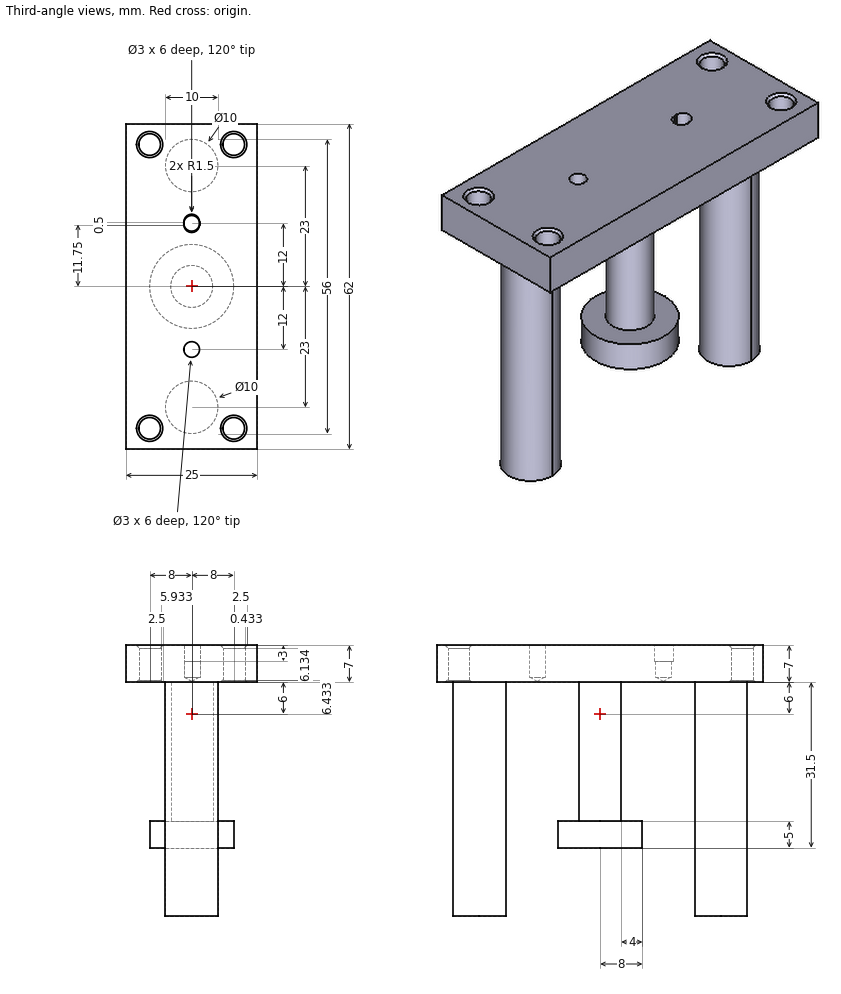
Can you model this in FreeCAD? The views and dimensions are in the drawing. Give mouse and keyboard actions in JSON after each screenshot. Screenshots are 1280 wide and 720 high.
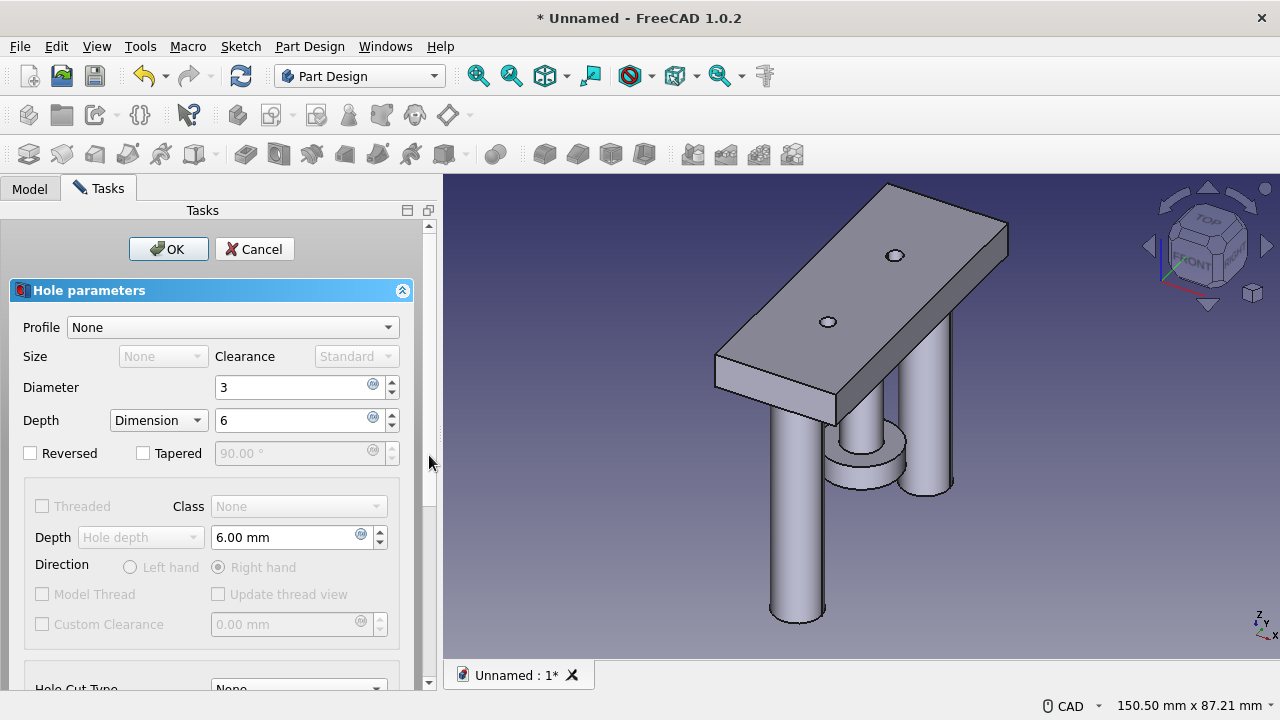
{"action": "left_click", "coordinate": [169, 249]}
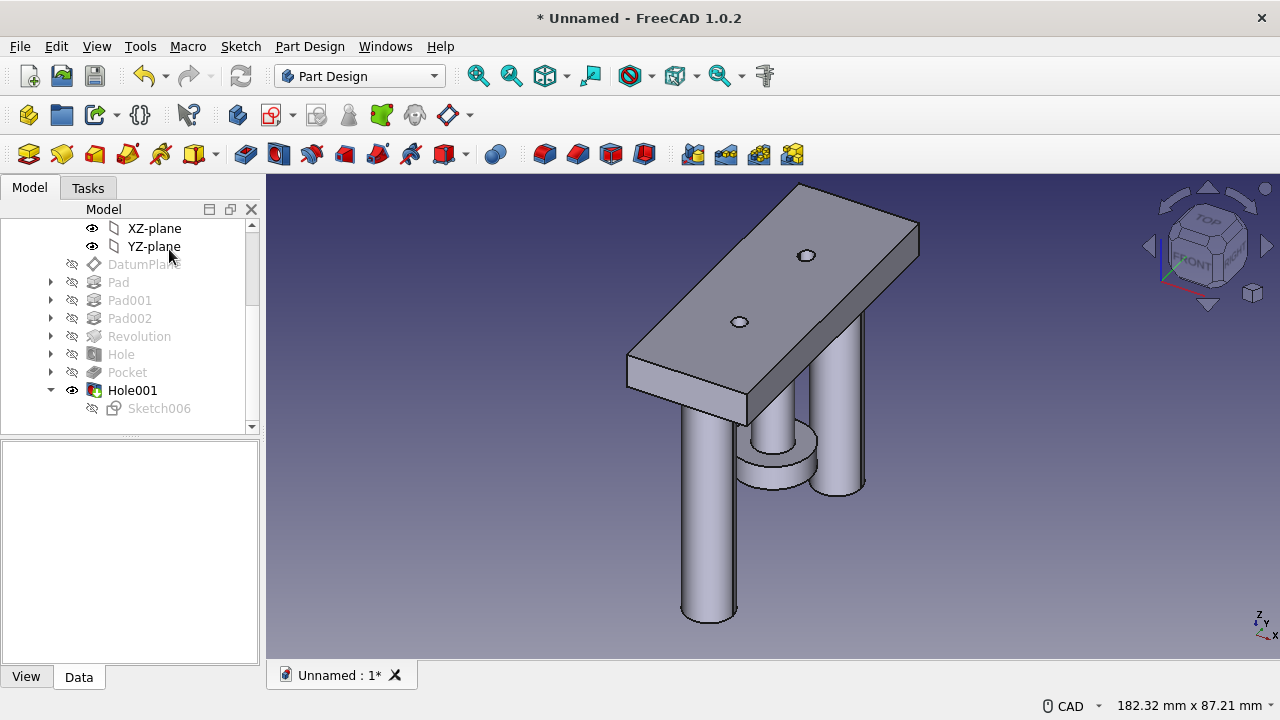
{"action": "scroll", "coordinate": [161, 314], "scroll_direction": "down", "scroll_amount": 3}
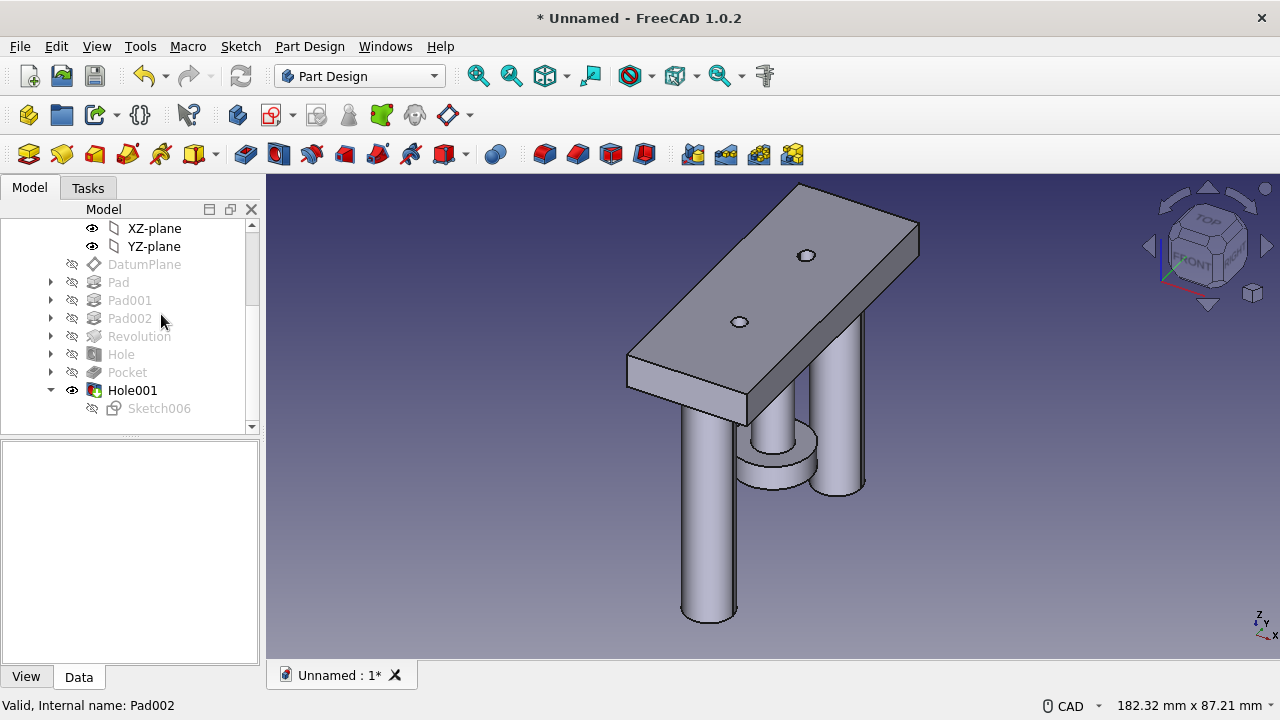
{"action": "scroll", "coordinate": [161, 314], "scroll_direction": "up", "scroll_amount": 15}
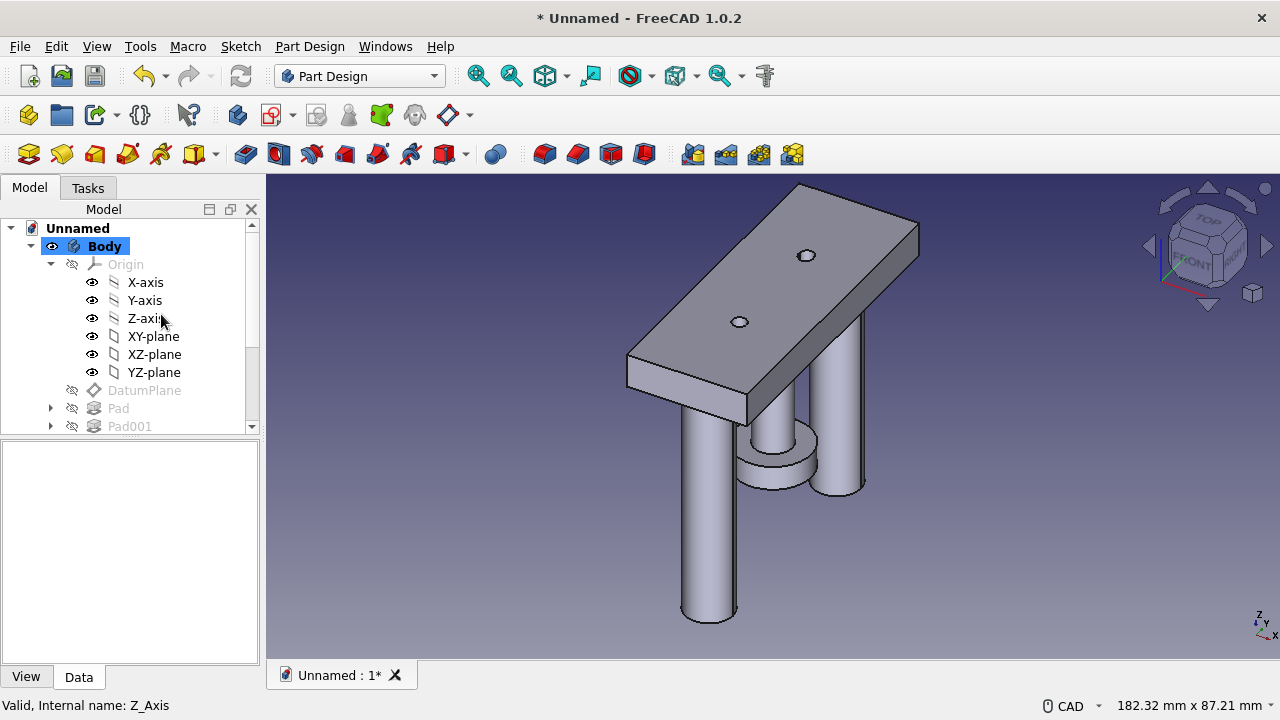
{"action": "left_click", "coordinate": [137, 354]}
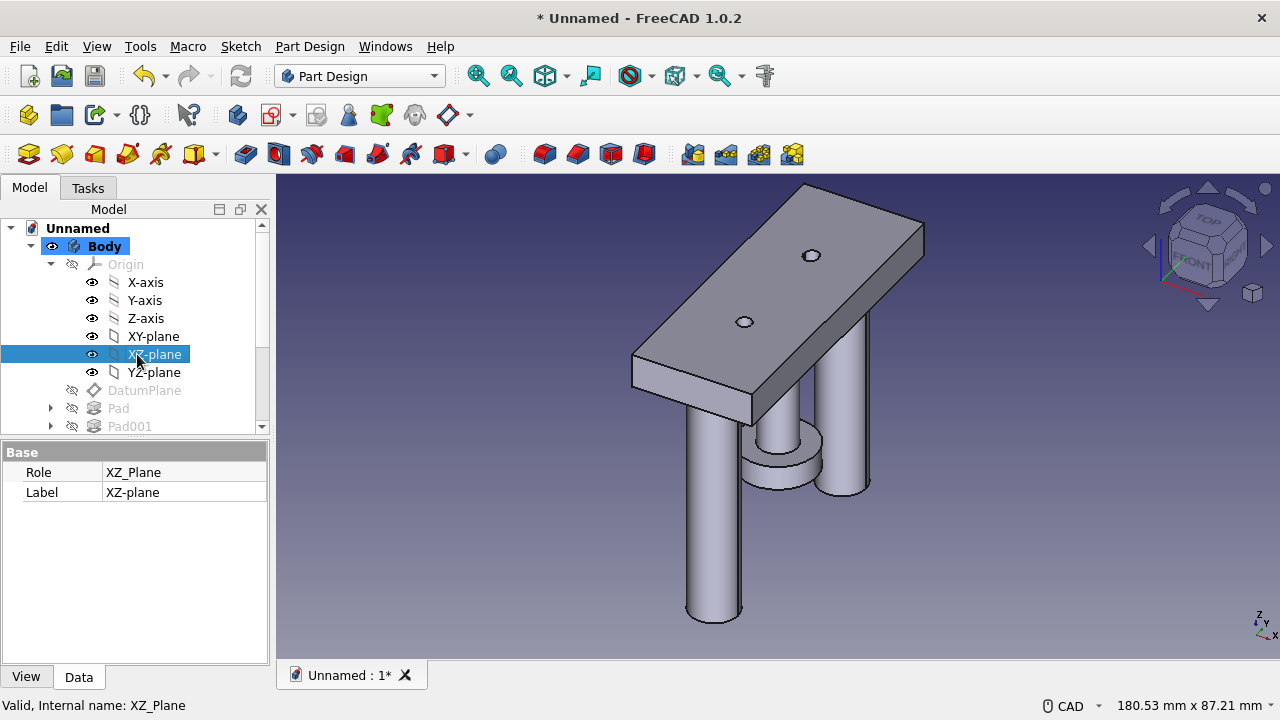
{"action": "left_click", "coordinate": [448, 116]}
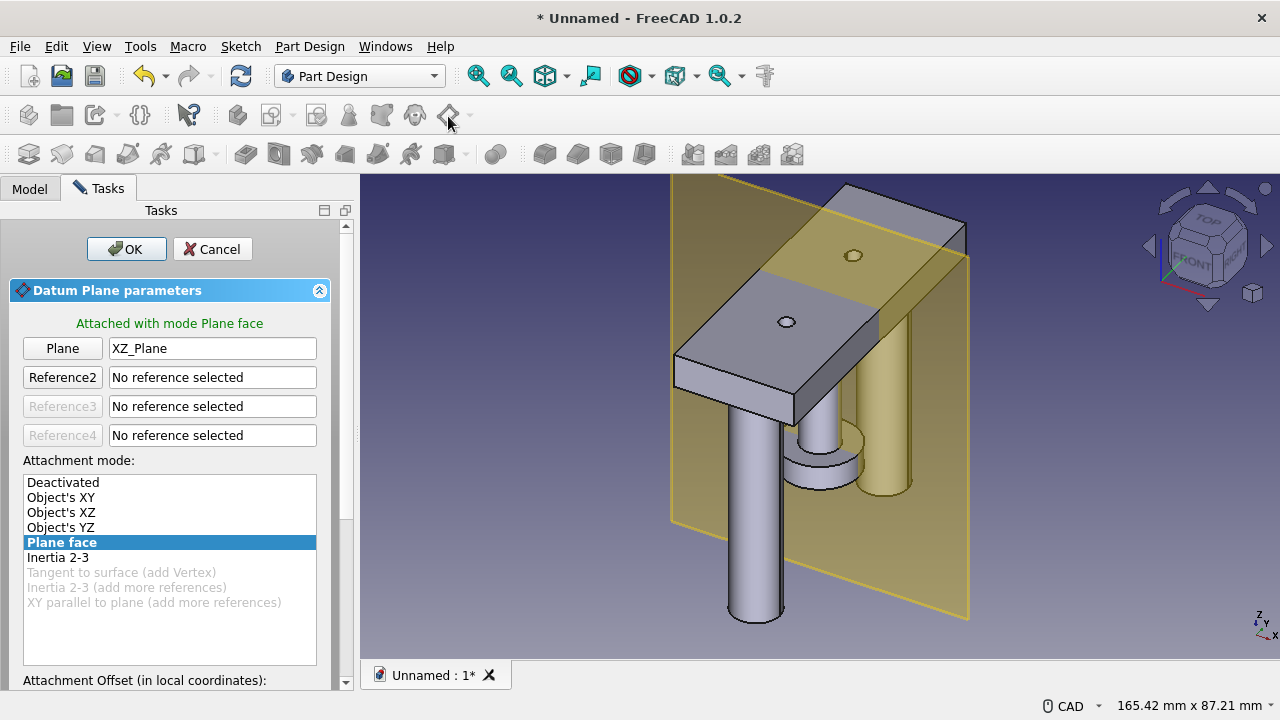
{"action": "scroll", "coordinate": [346, 455], "scroll_direction": "down", "scroll_amount": 3}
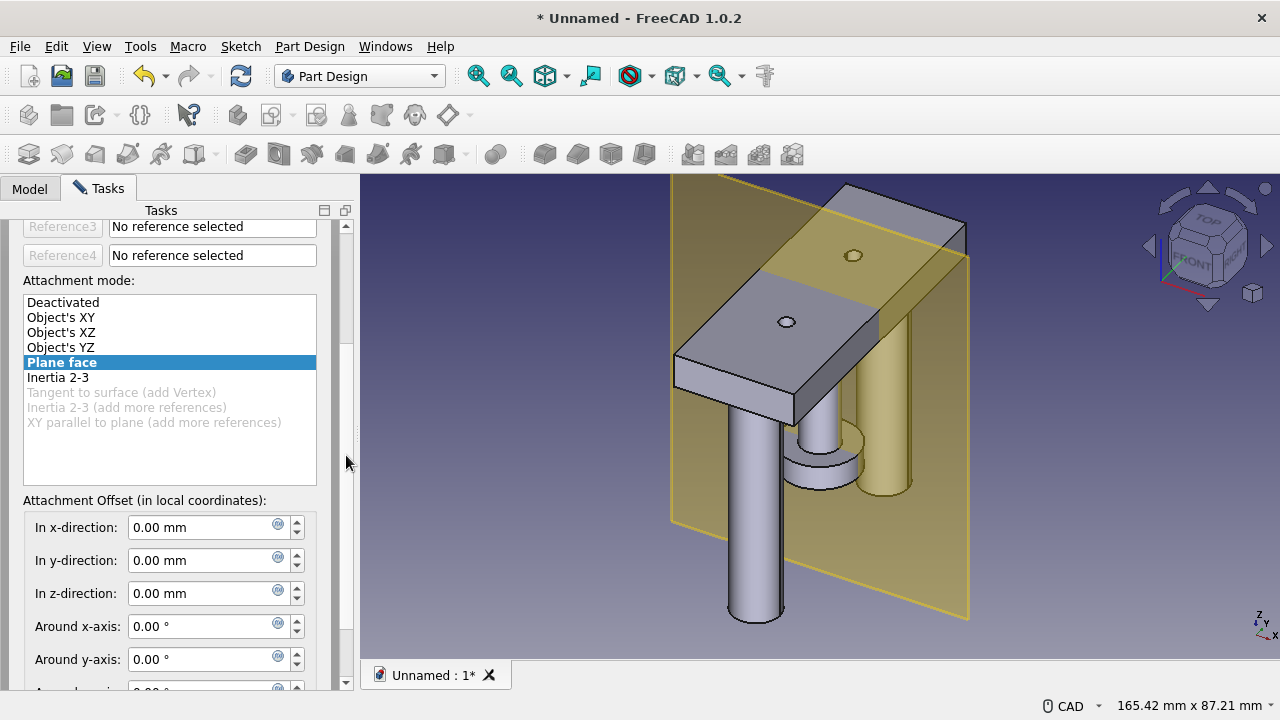
{"action": "triple_click", "coordinate": [210, 594]}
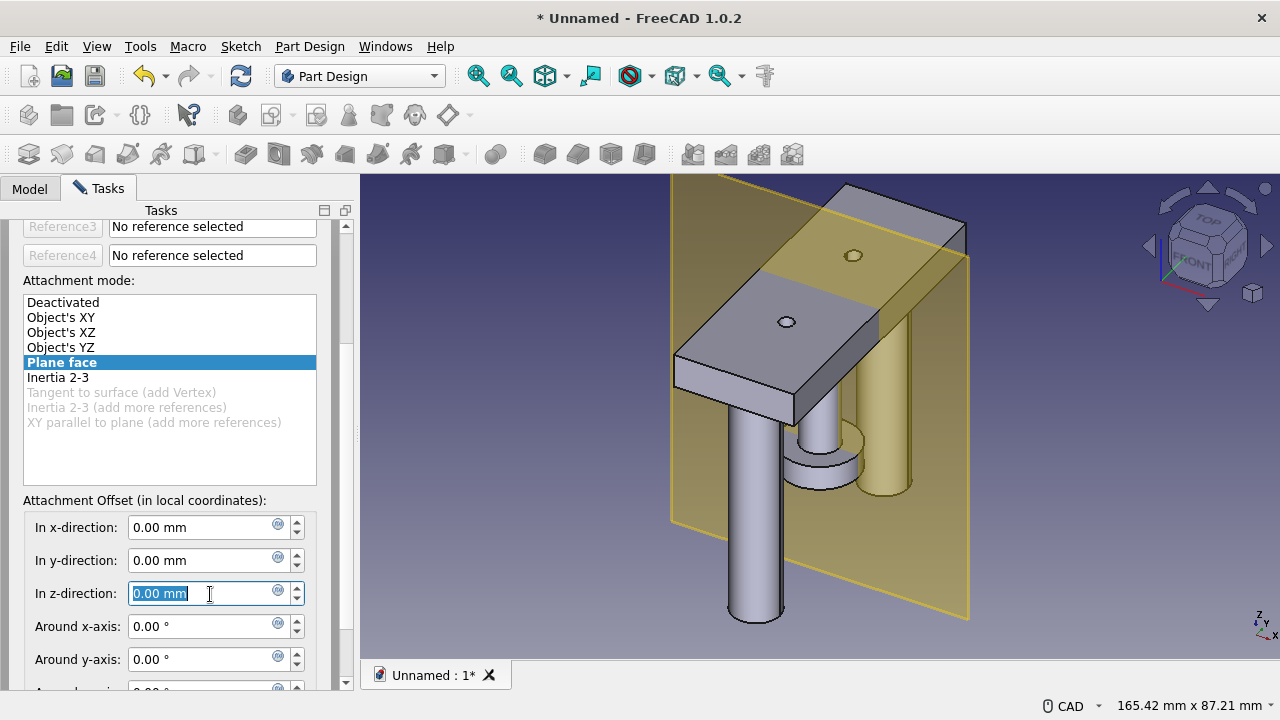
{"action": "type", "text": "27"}
{"action": "key", "text": "Tab"}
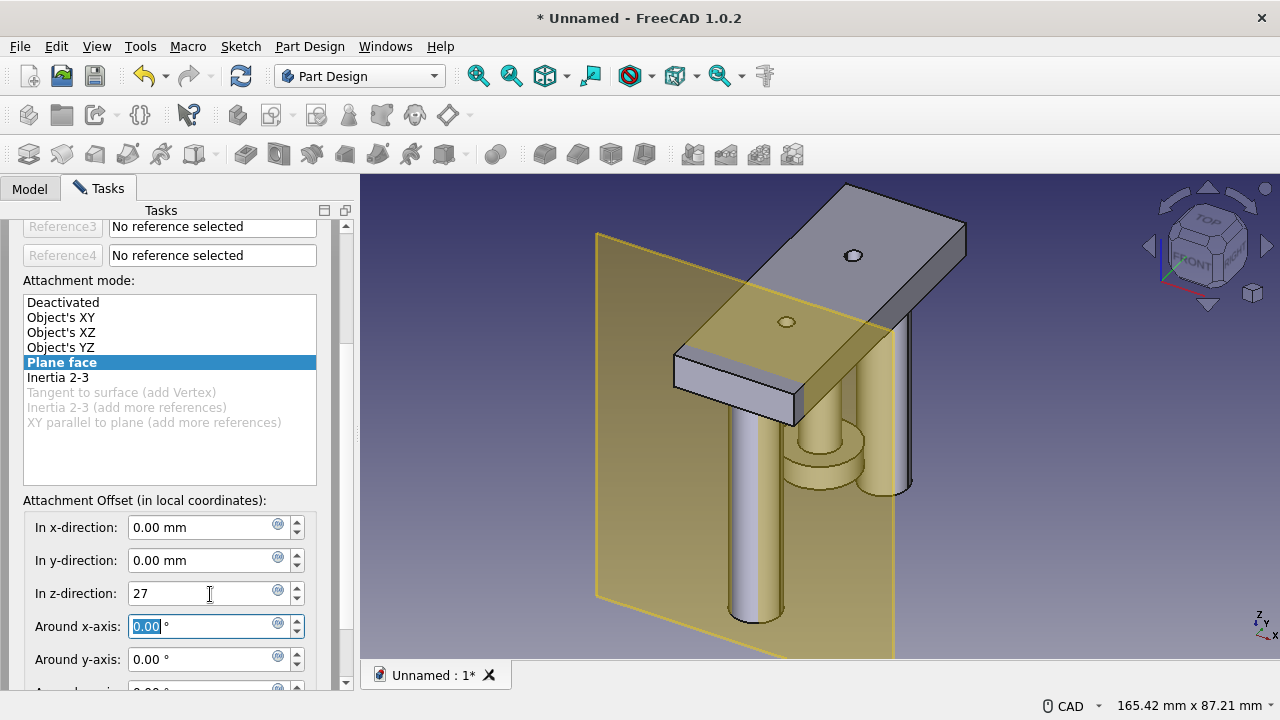
{"action": "scroll", "coordinate": [346, 455], "scroll_direction": "up", "scroll_amount": 4}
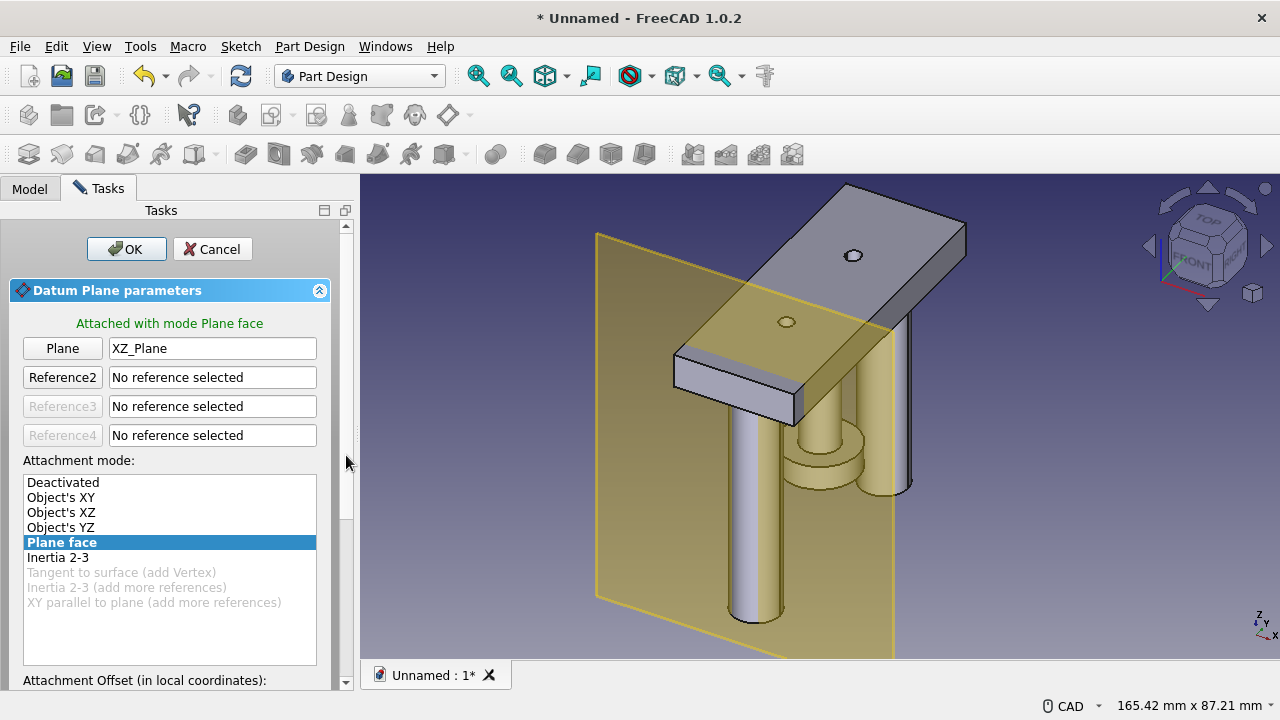
{"action": "left_click", "coordinate": [127, 249]}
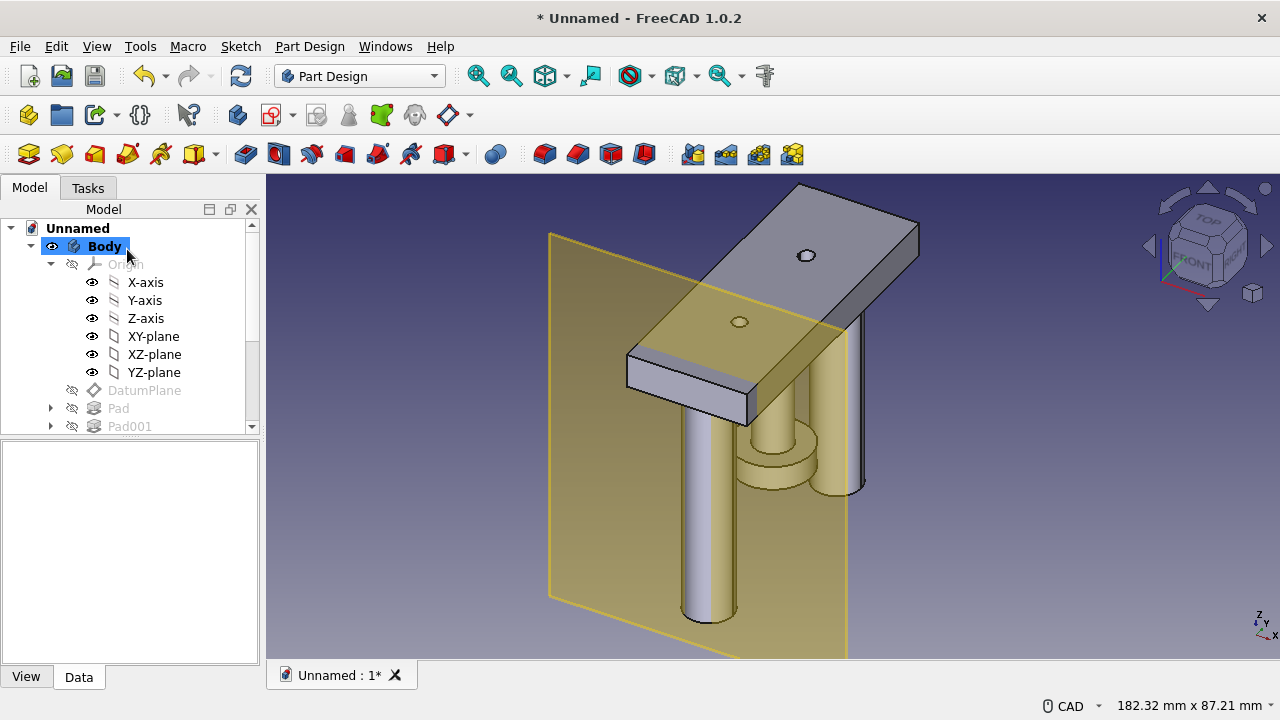
{"action": "scroll", "coordinate": [101, 332], "scroll_direction": "down", "scroll_amount": 3}